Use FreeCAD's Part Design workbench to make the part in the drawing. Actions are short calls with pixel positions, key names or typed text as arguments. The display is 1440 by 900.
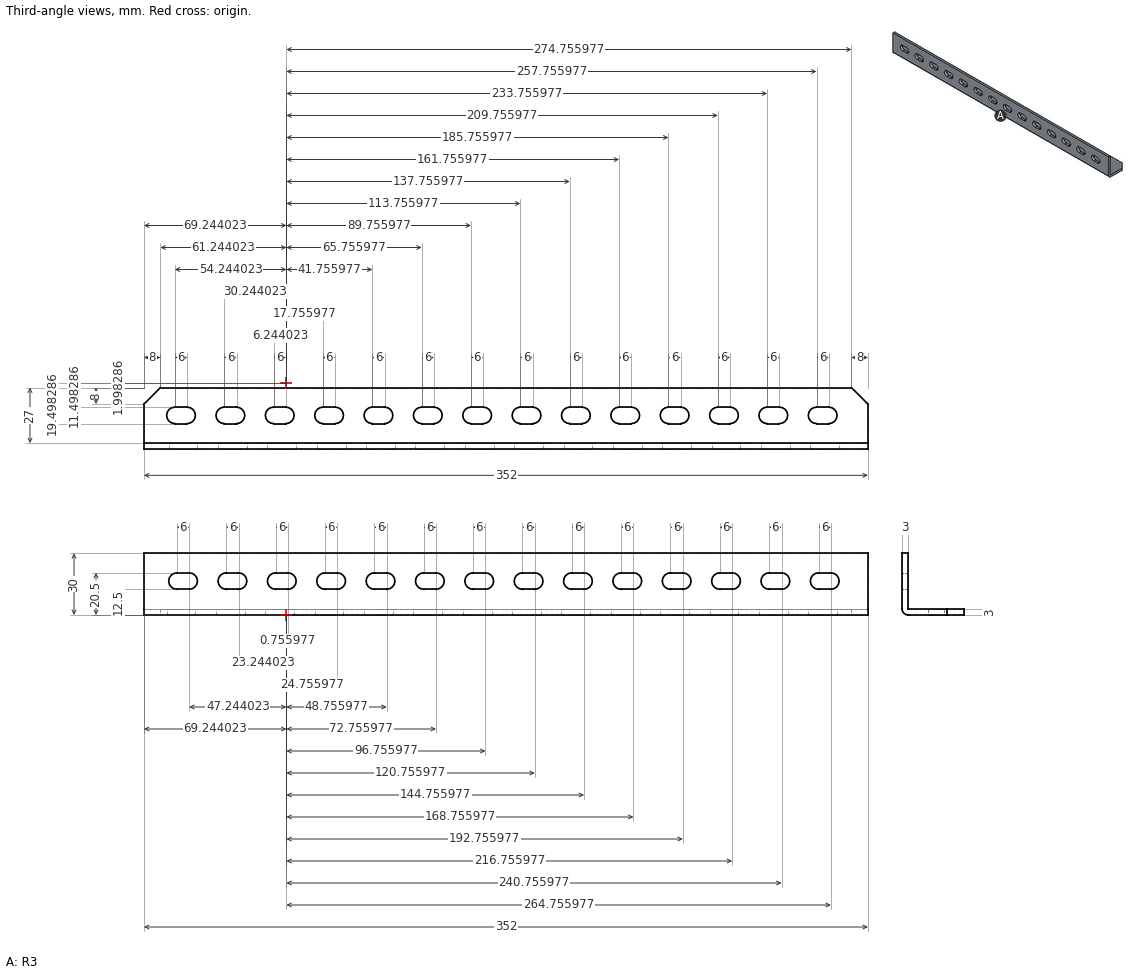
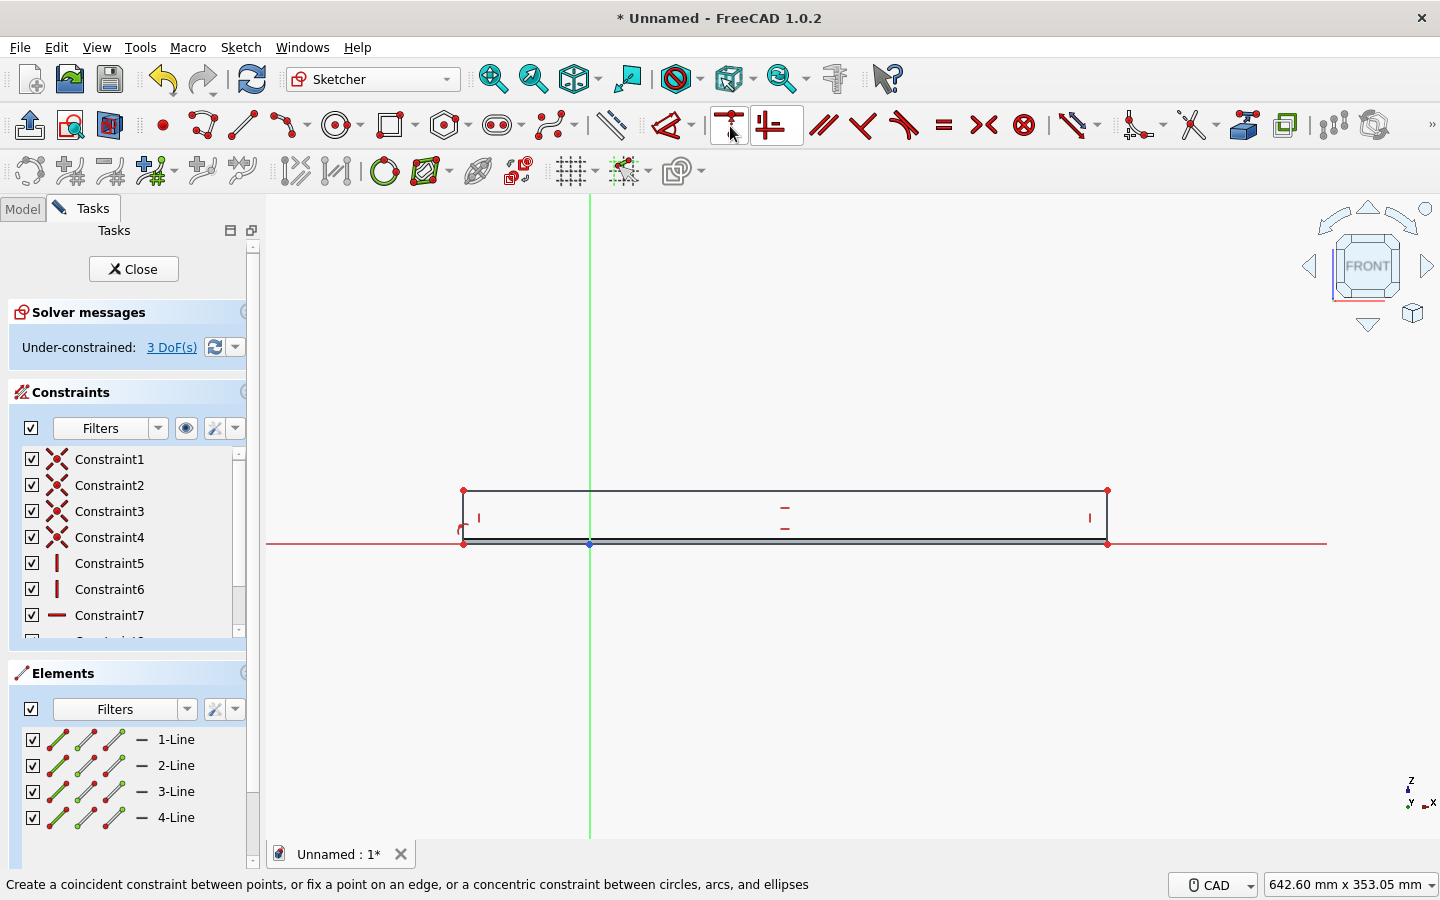
click(666, 126)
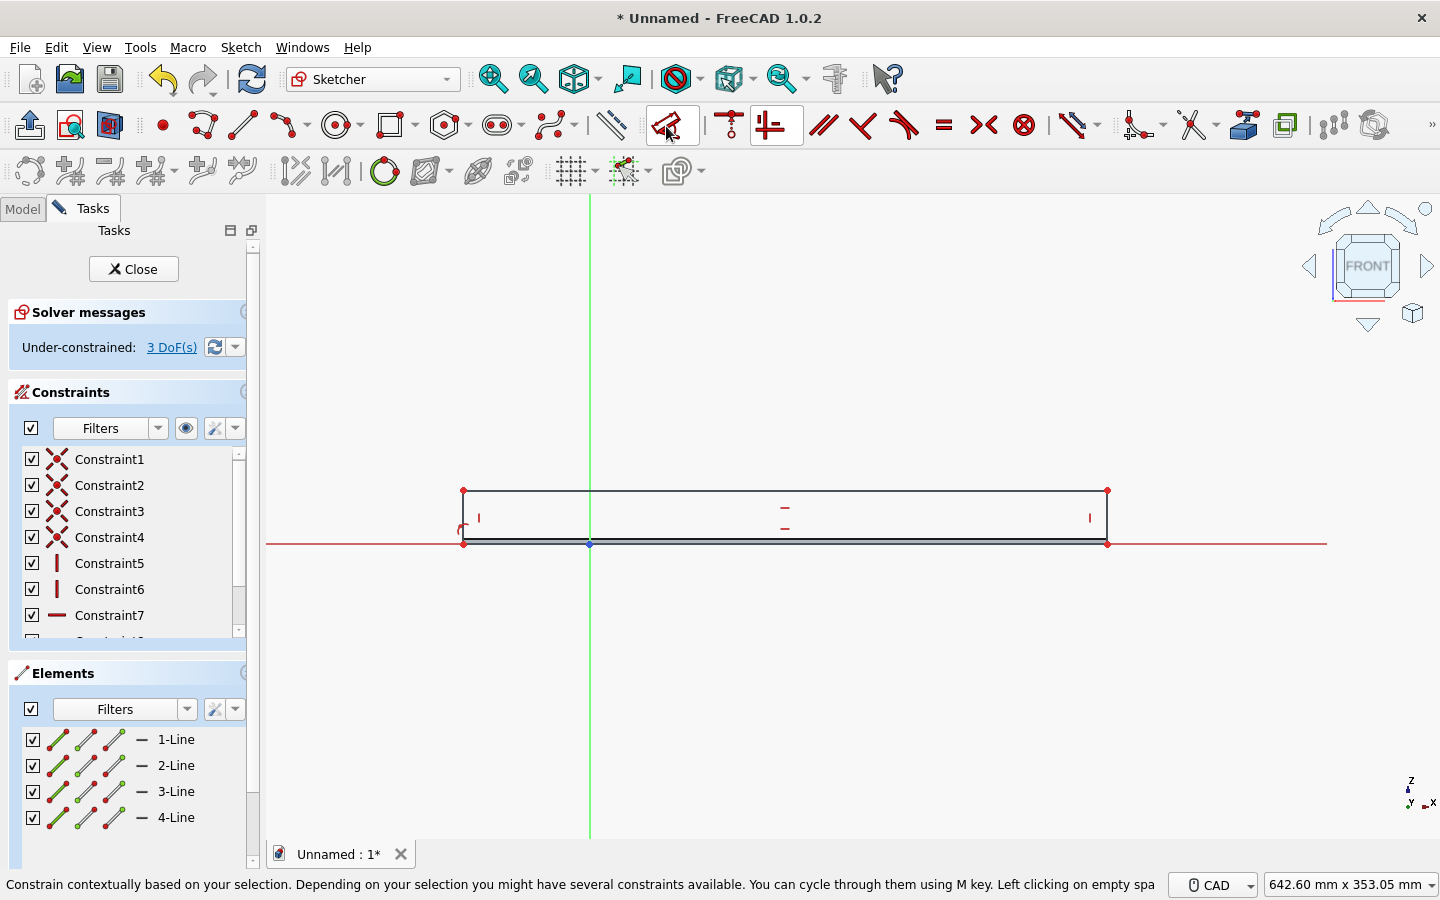
click(463, 507)
click(429, 518)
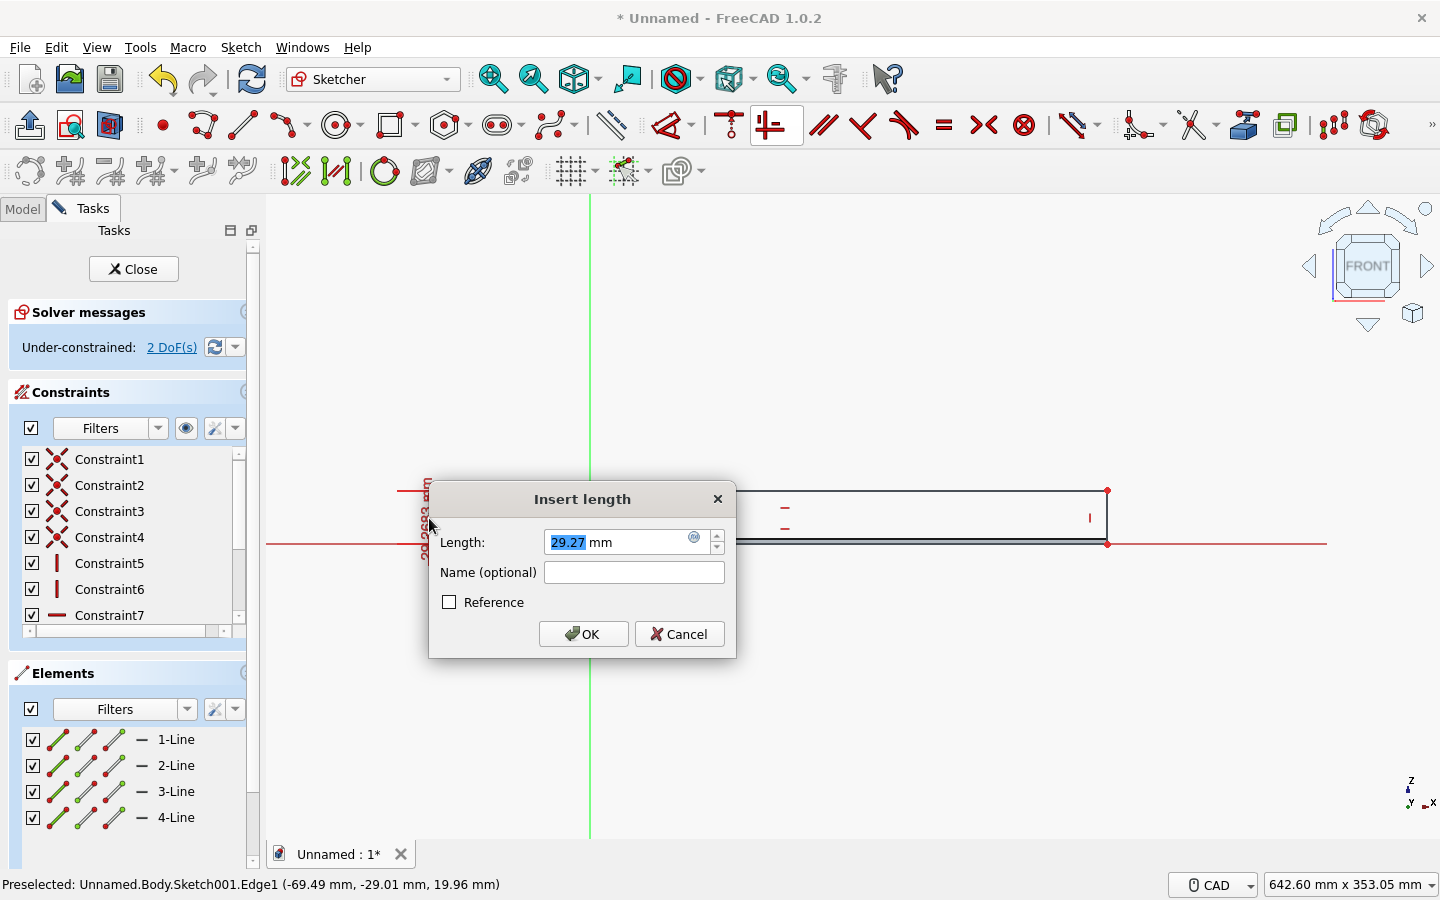
text(30)
key(Return)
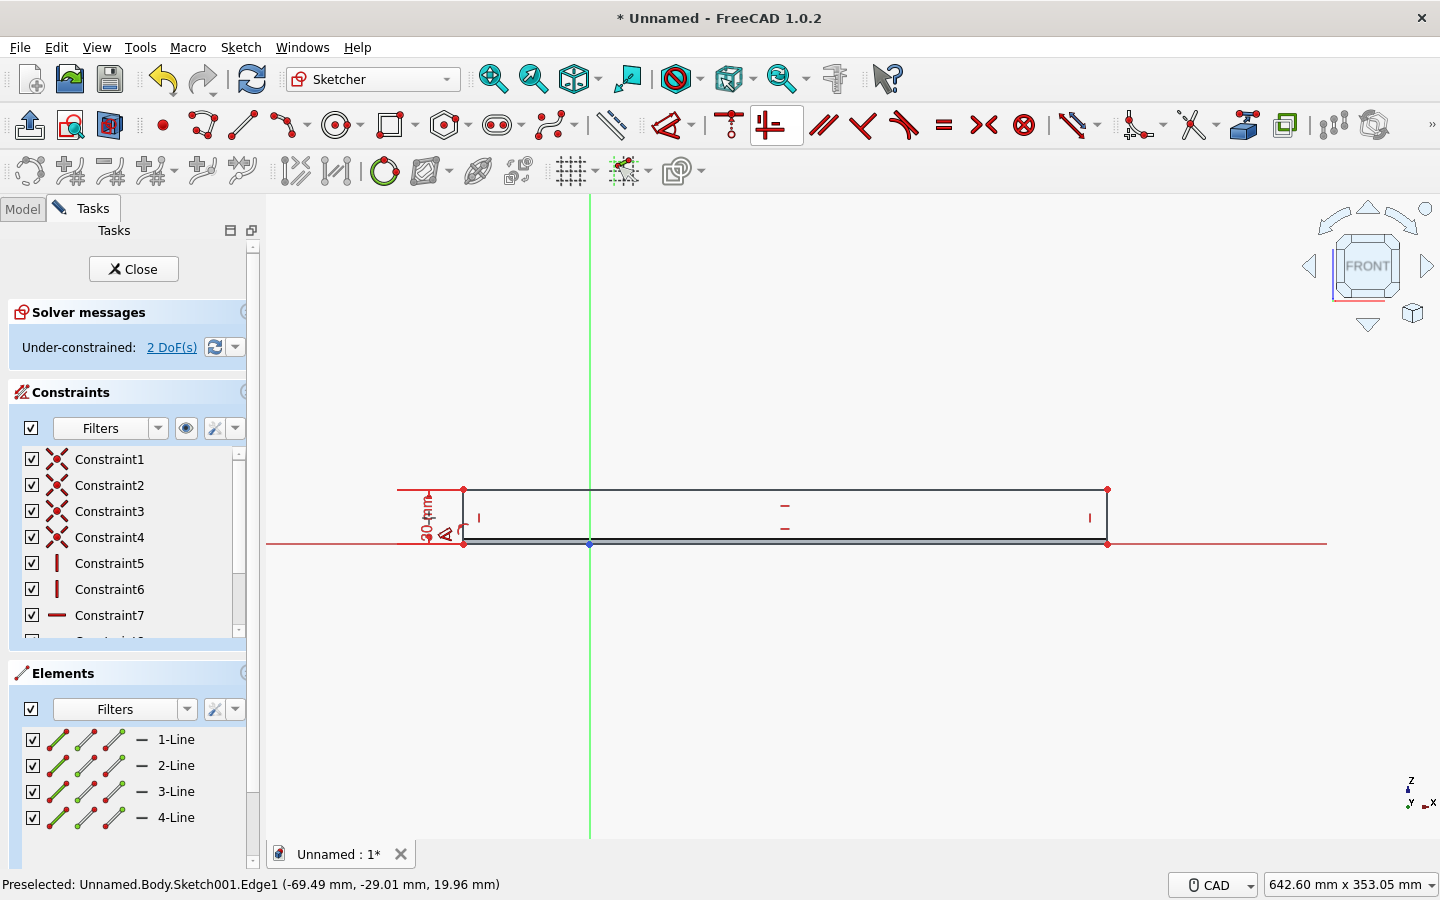
click(656, 544)
click(785, 578)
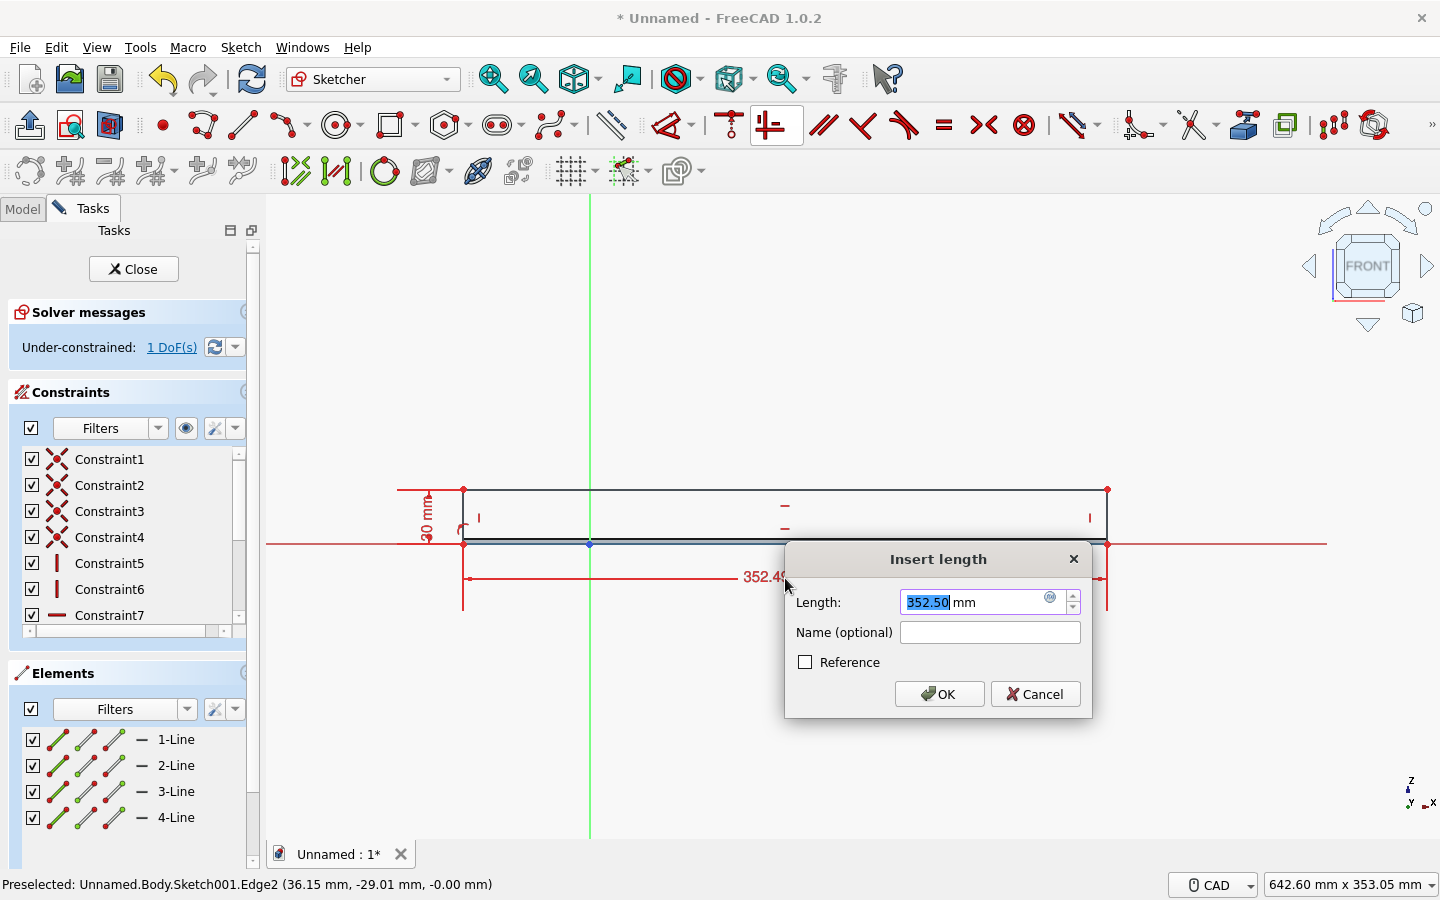
text(352)
key(Return)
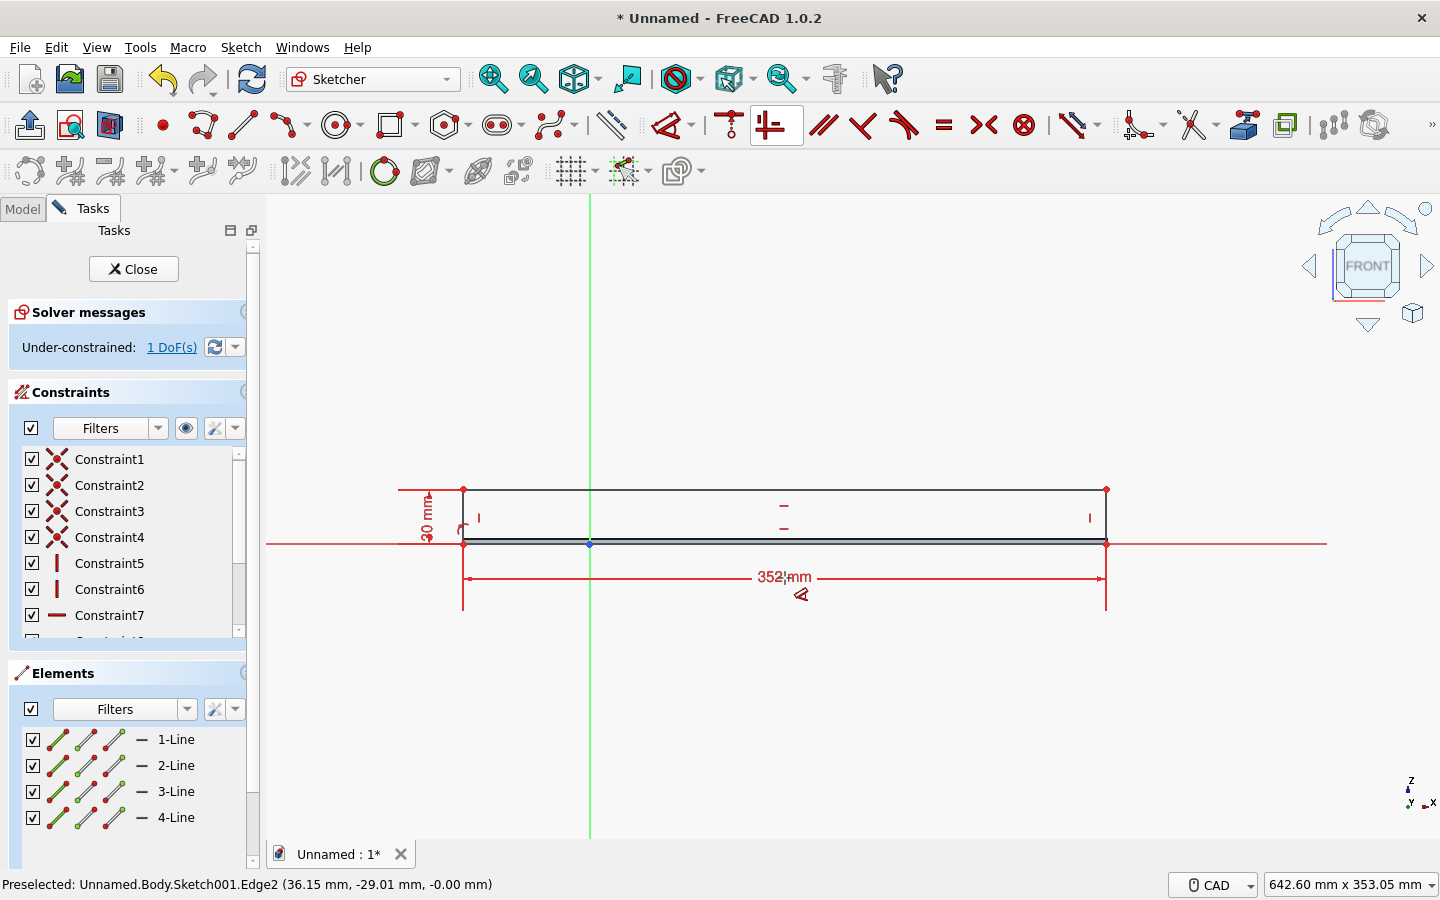
click(463, 490)
click(527, 578)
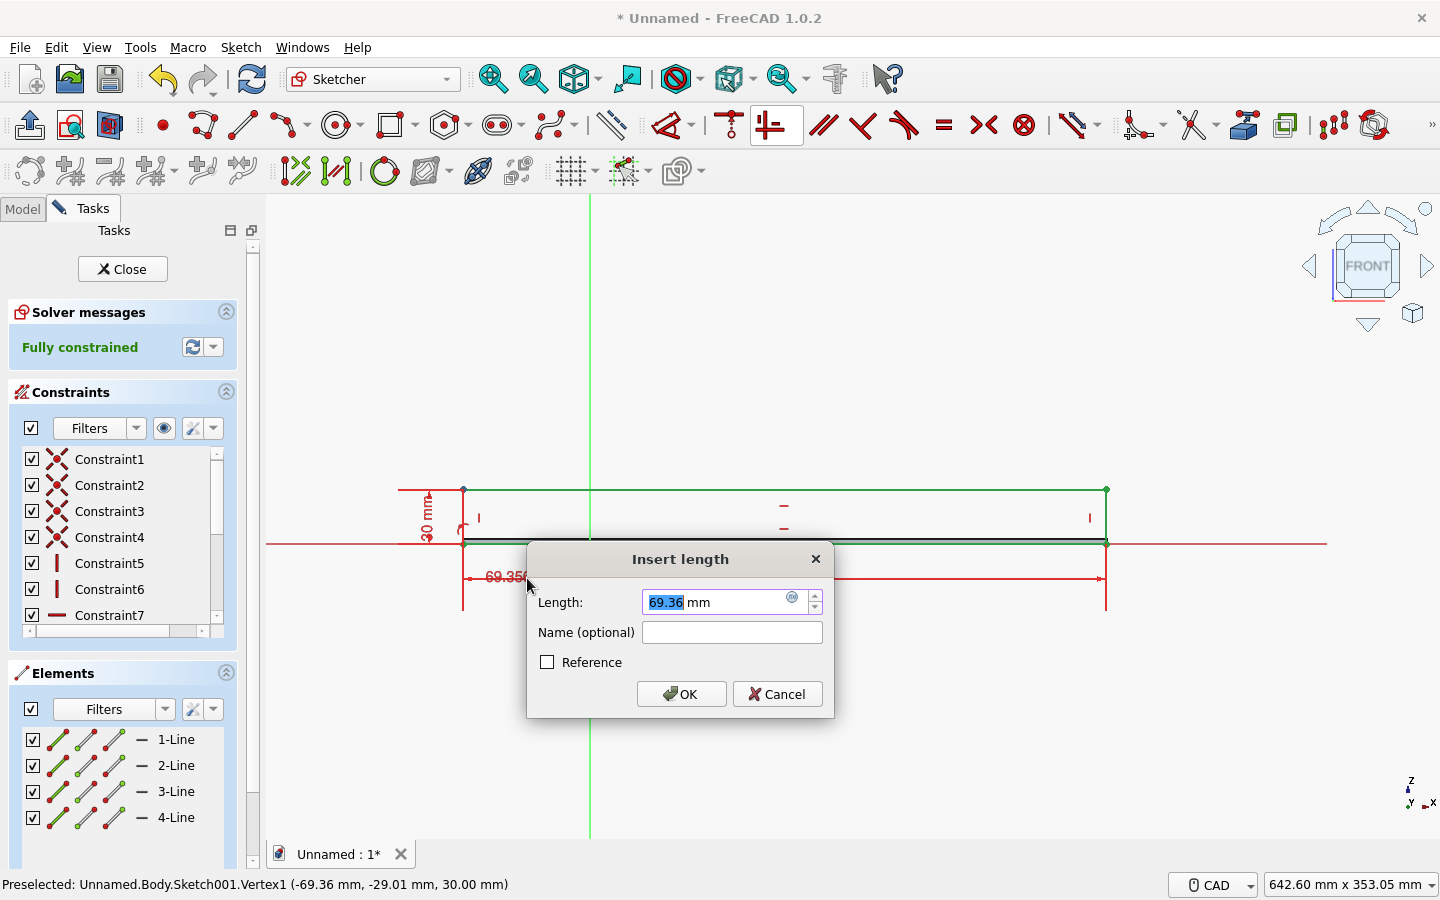
text(69.244023)
key(Return)
key(Escape)